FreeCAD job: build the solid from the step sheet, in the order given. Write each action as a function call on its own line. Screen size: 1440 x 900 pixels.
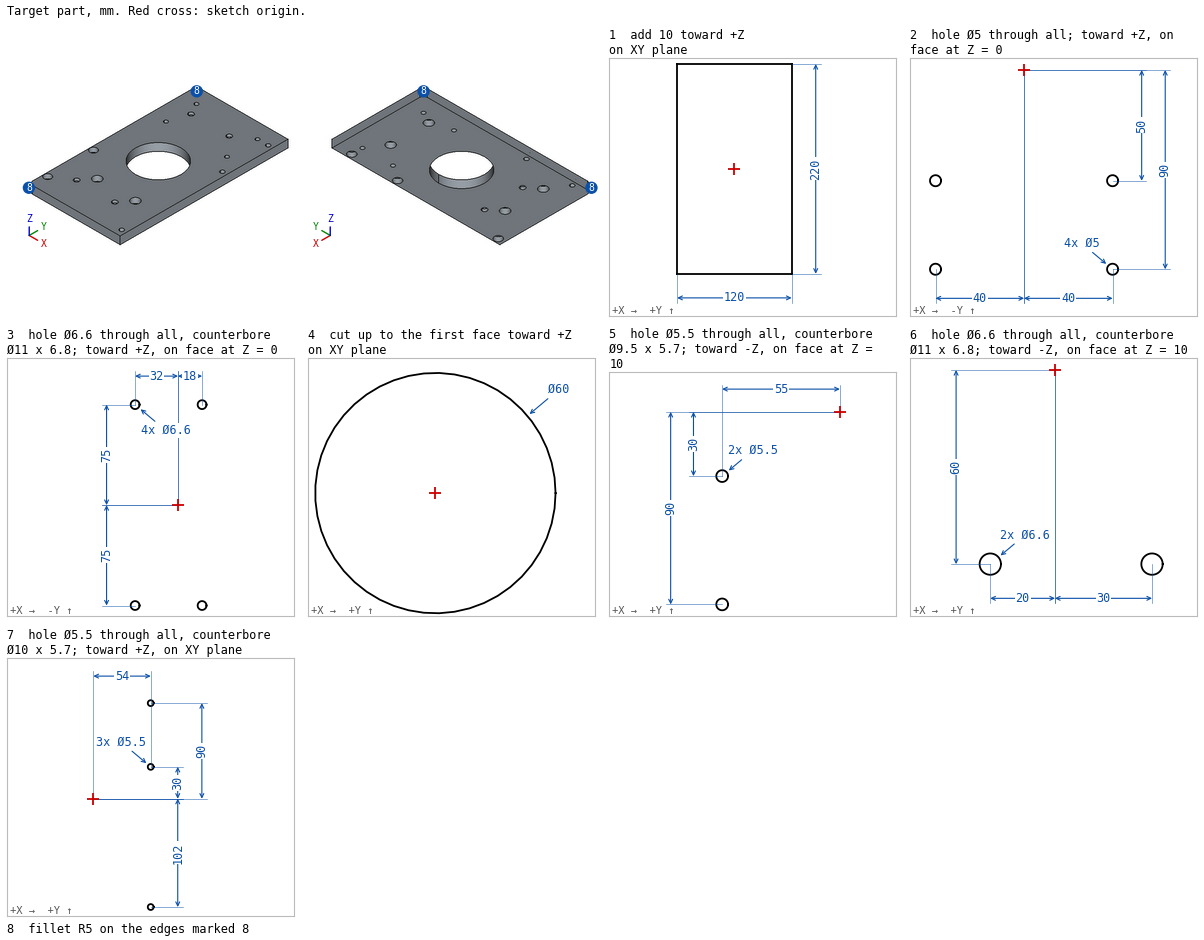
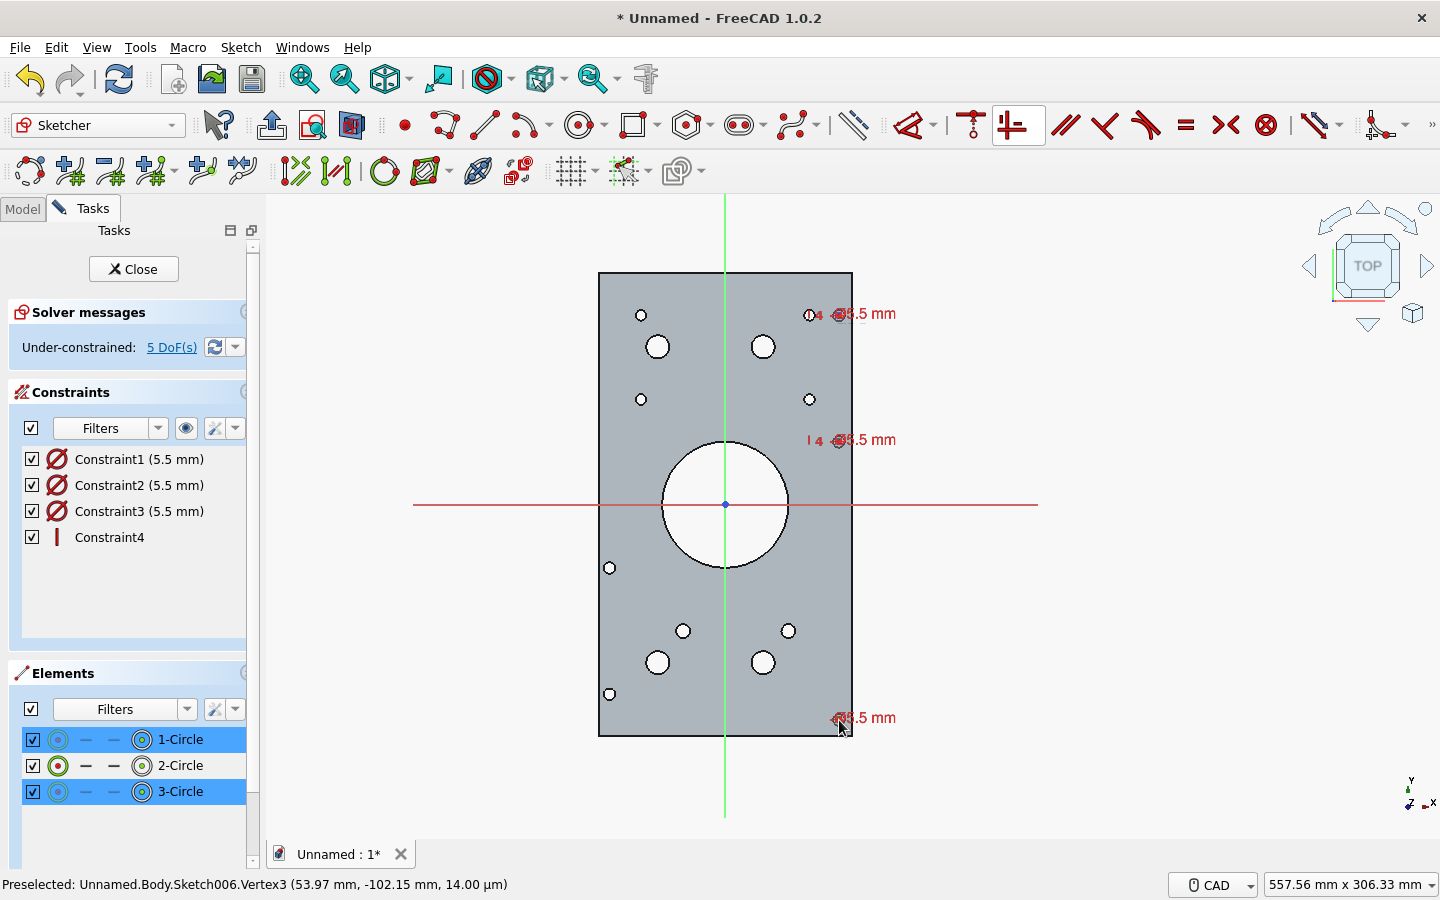
key(v)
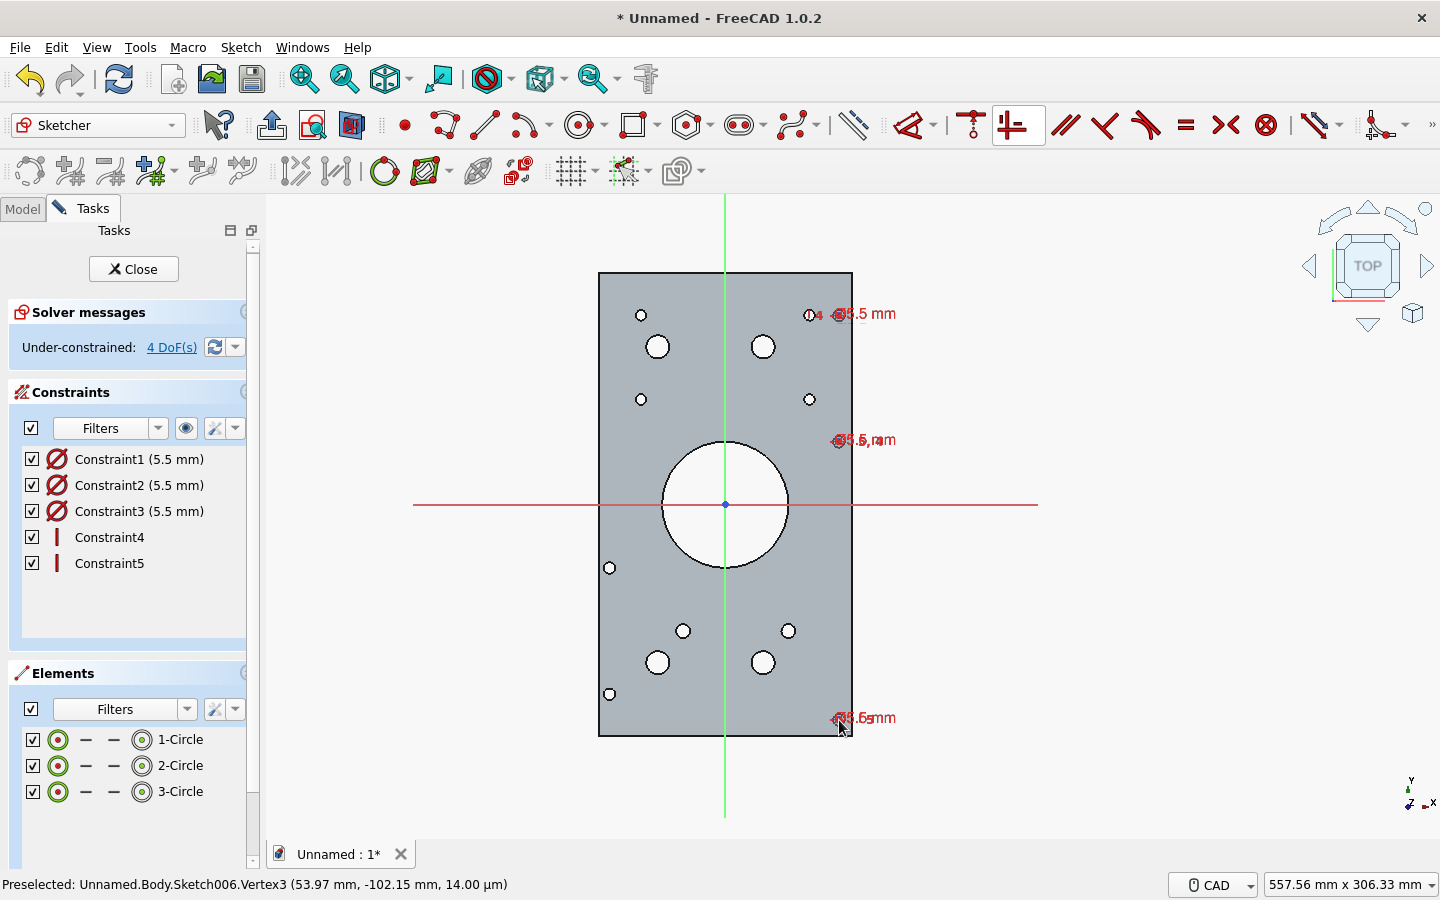
click(908, 126)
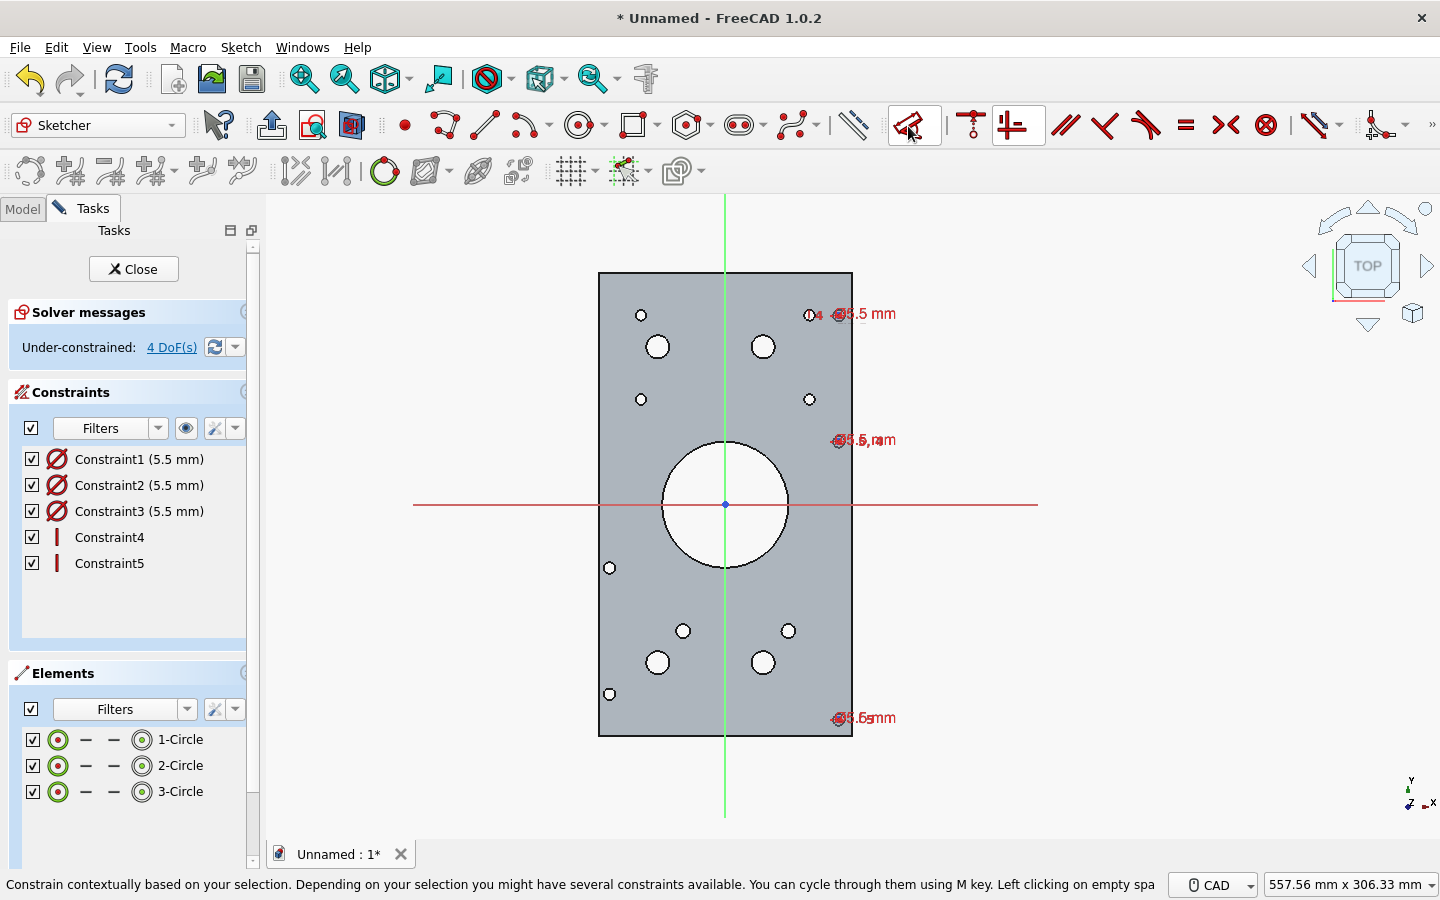
click(839, 442)
click(782, 408)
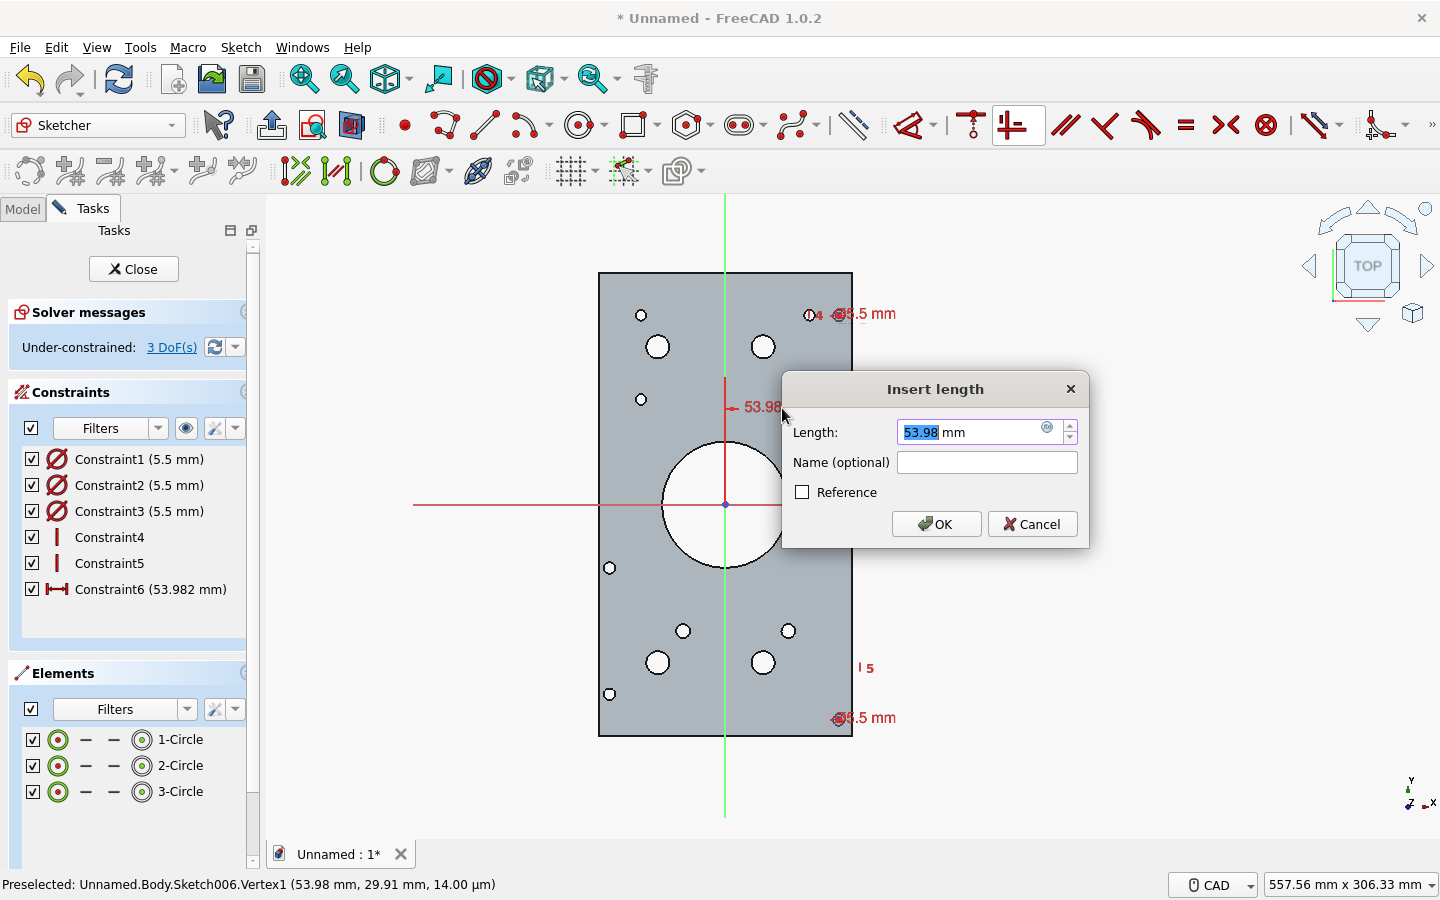
text(54)
key(Return)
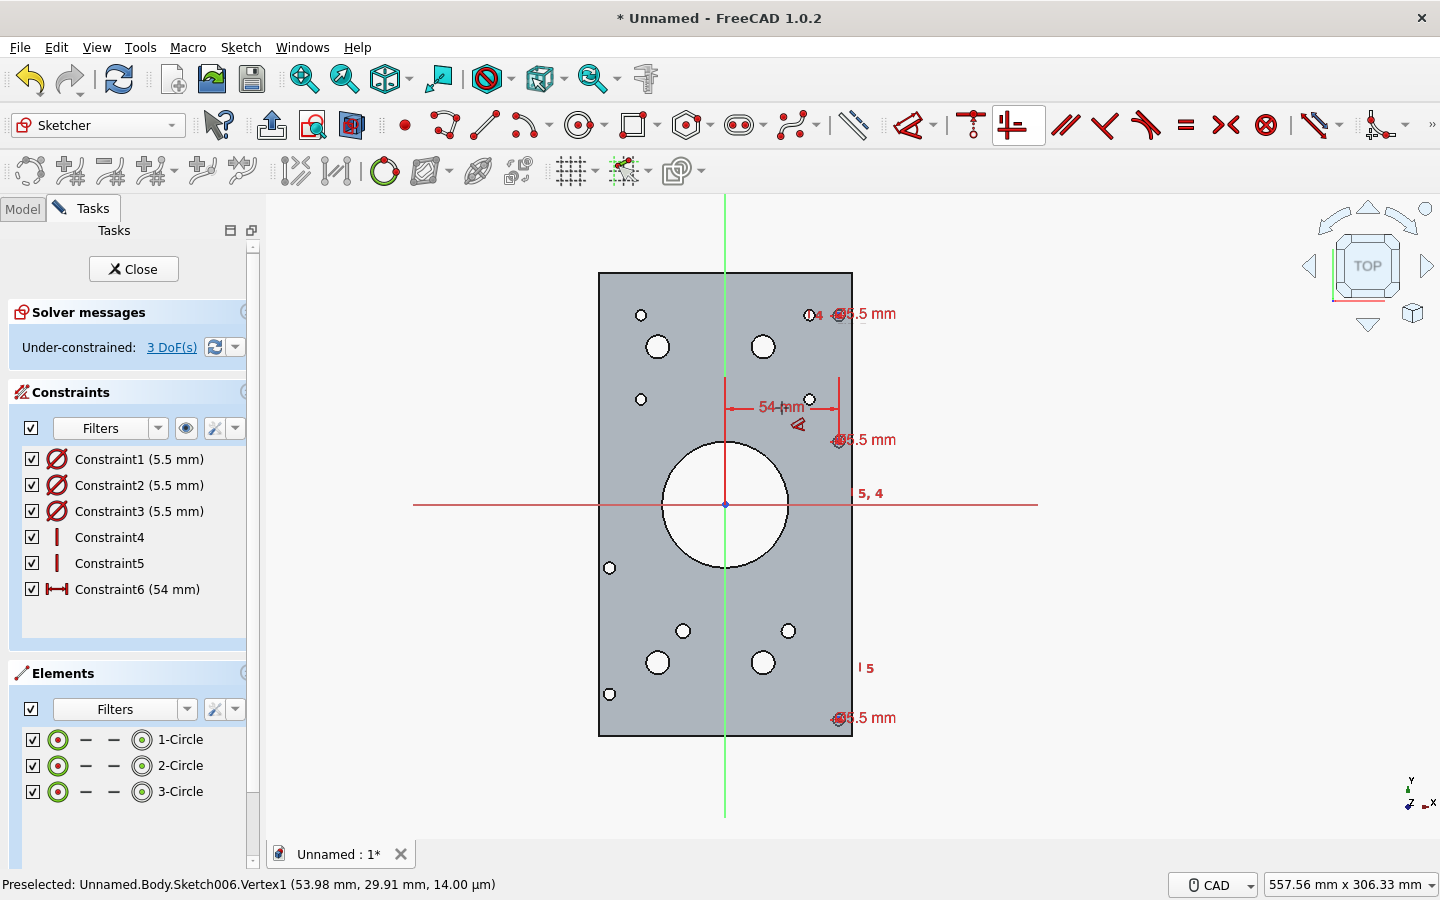
click(839, 442)
click(691, 473)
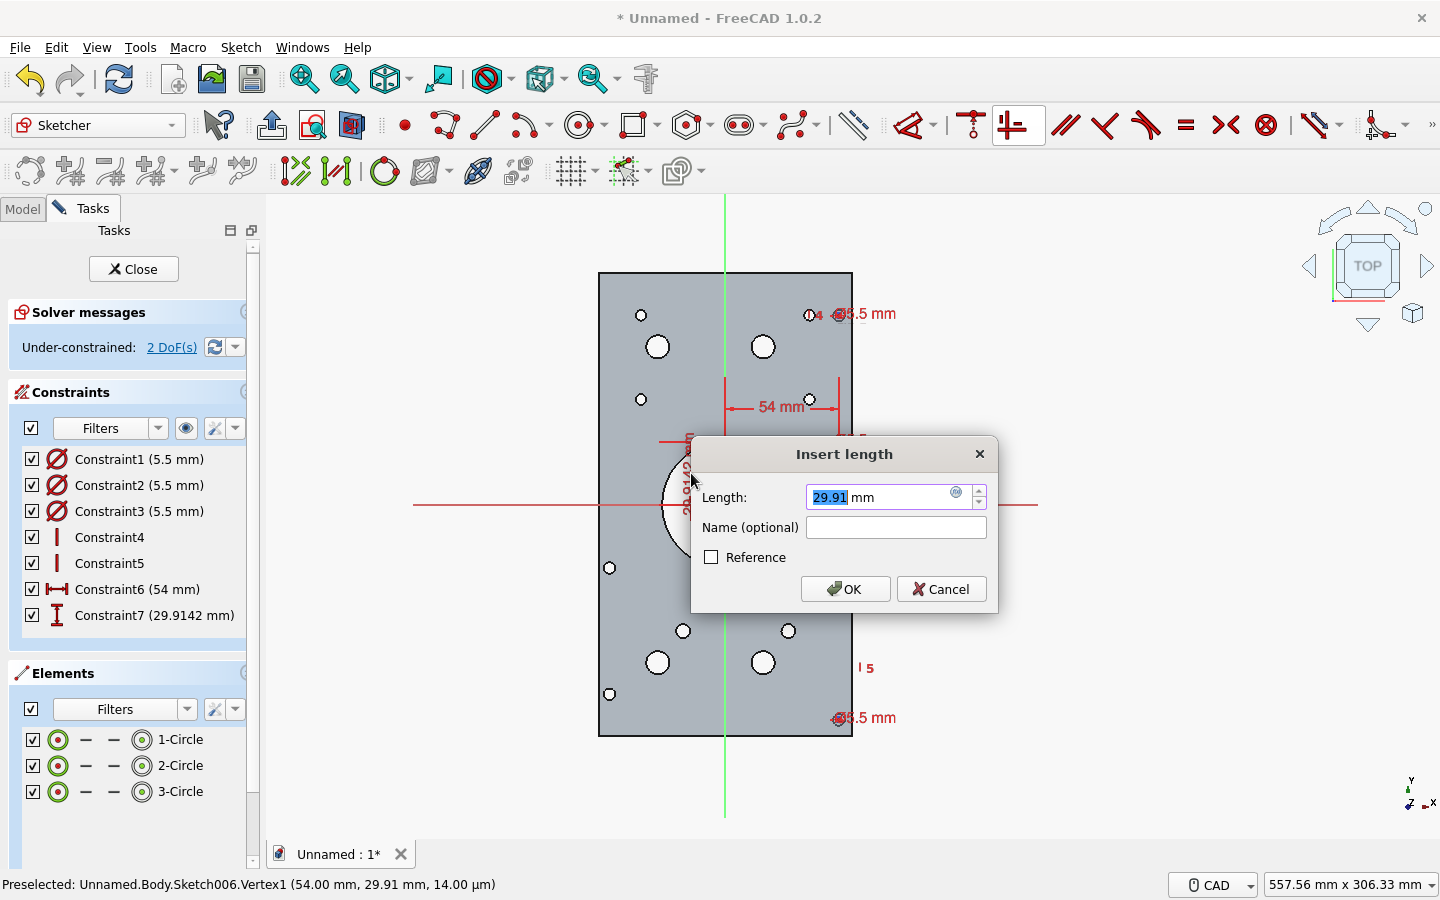
text(30)
key(Return)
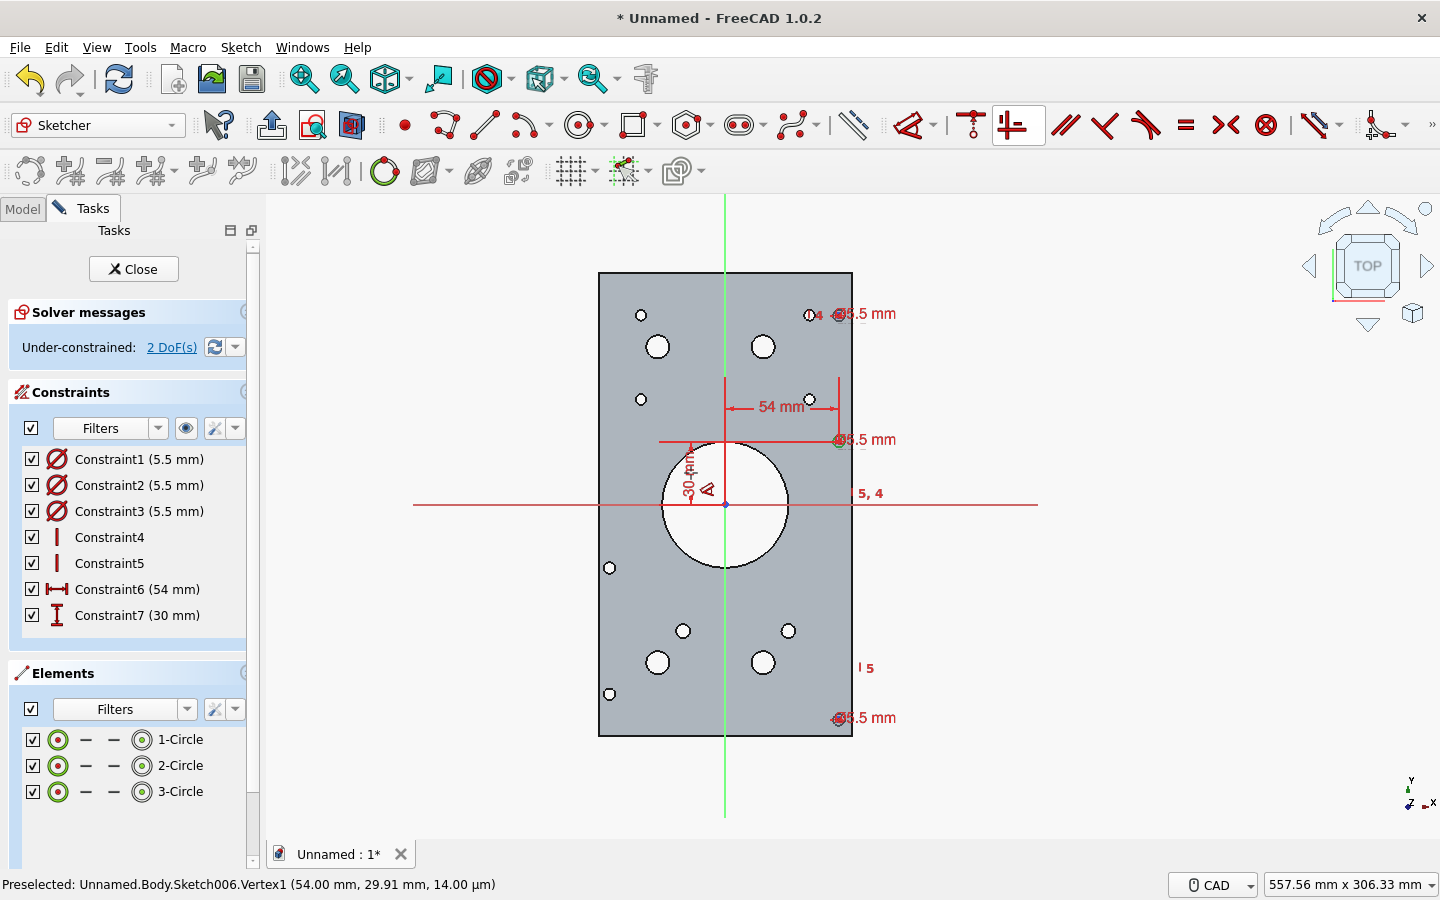
click(839, 316)
click(691, 410)